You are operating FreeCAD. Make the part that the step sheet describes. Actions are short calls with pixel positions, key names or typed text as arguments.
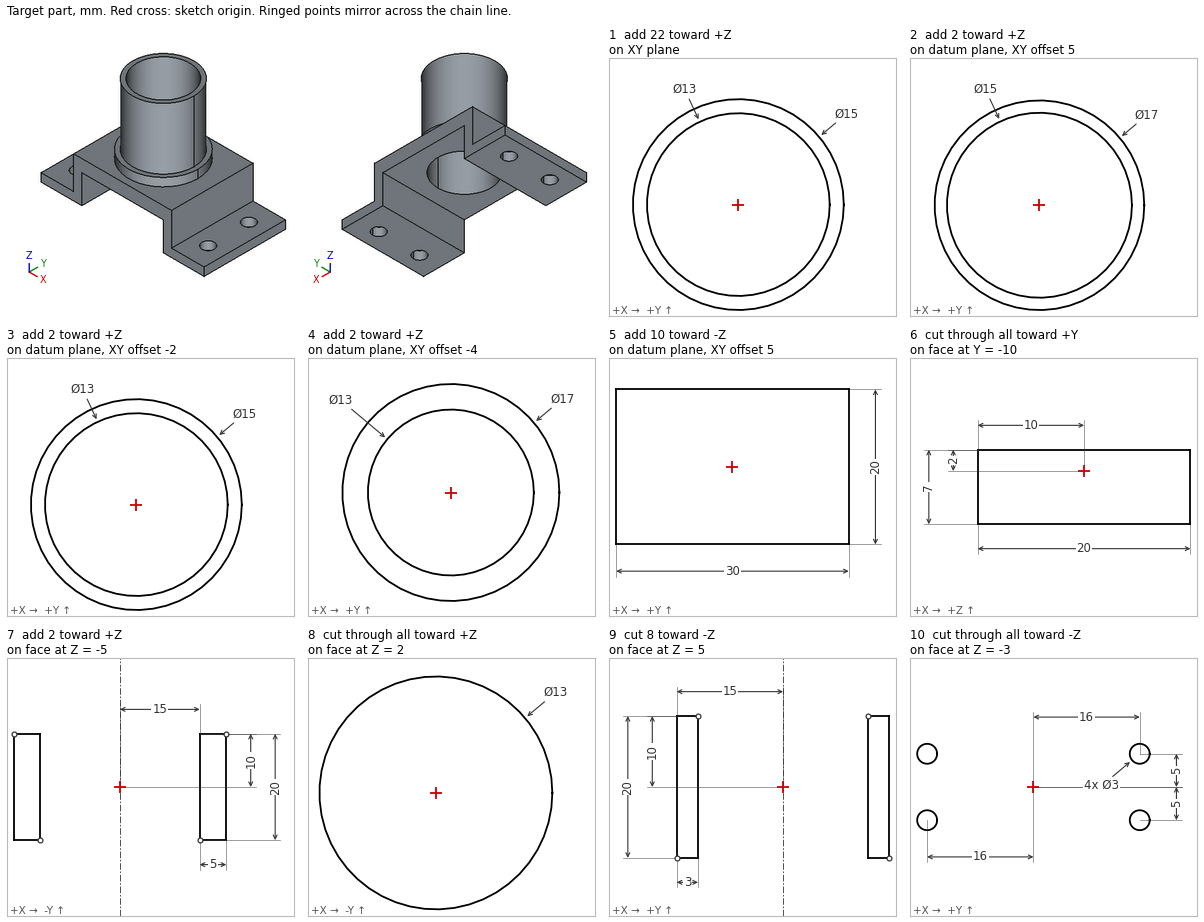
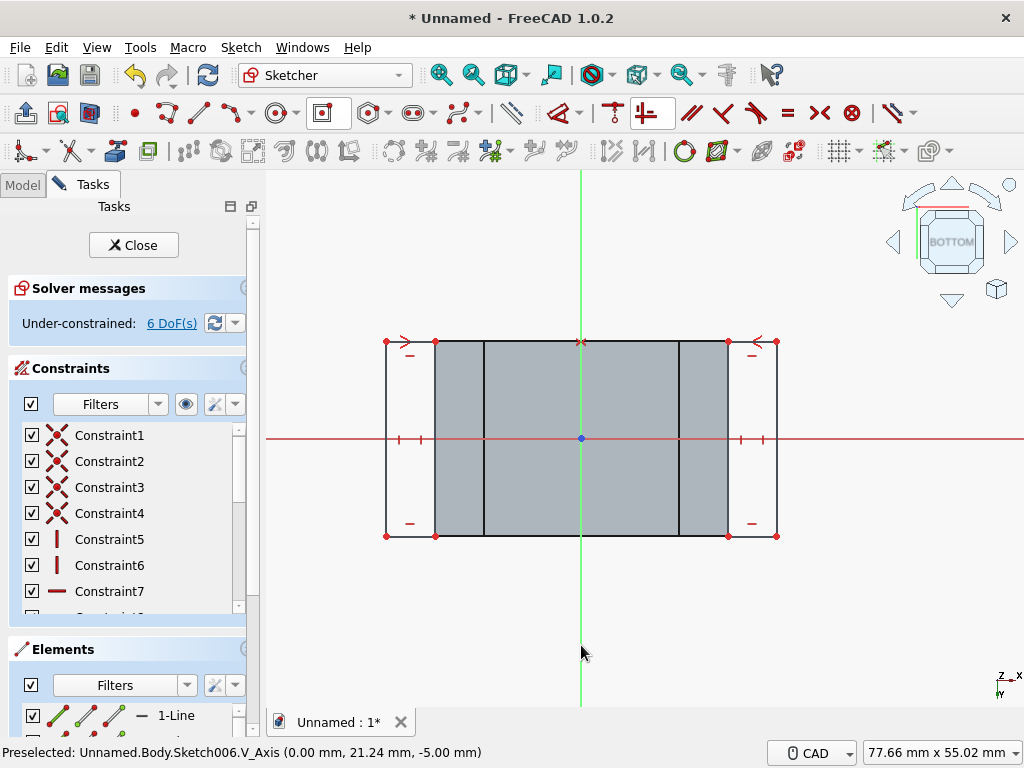
click(728, 537)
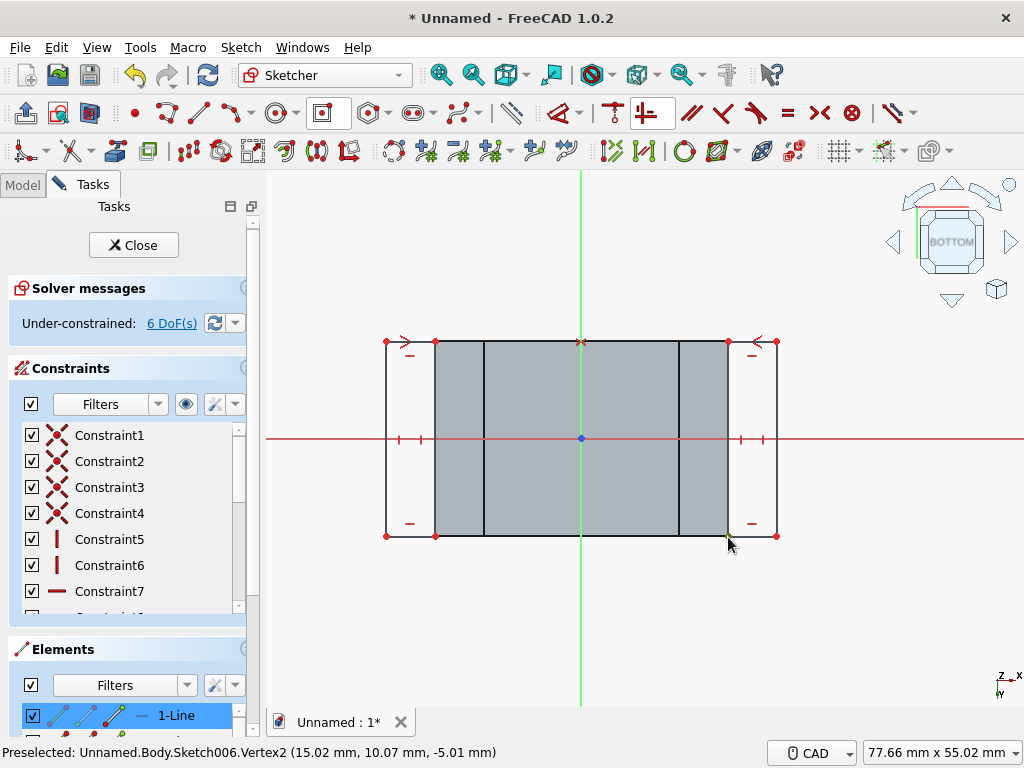
click(435, 537)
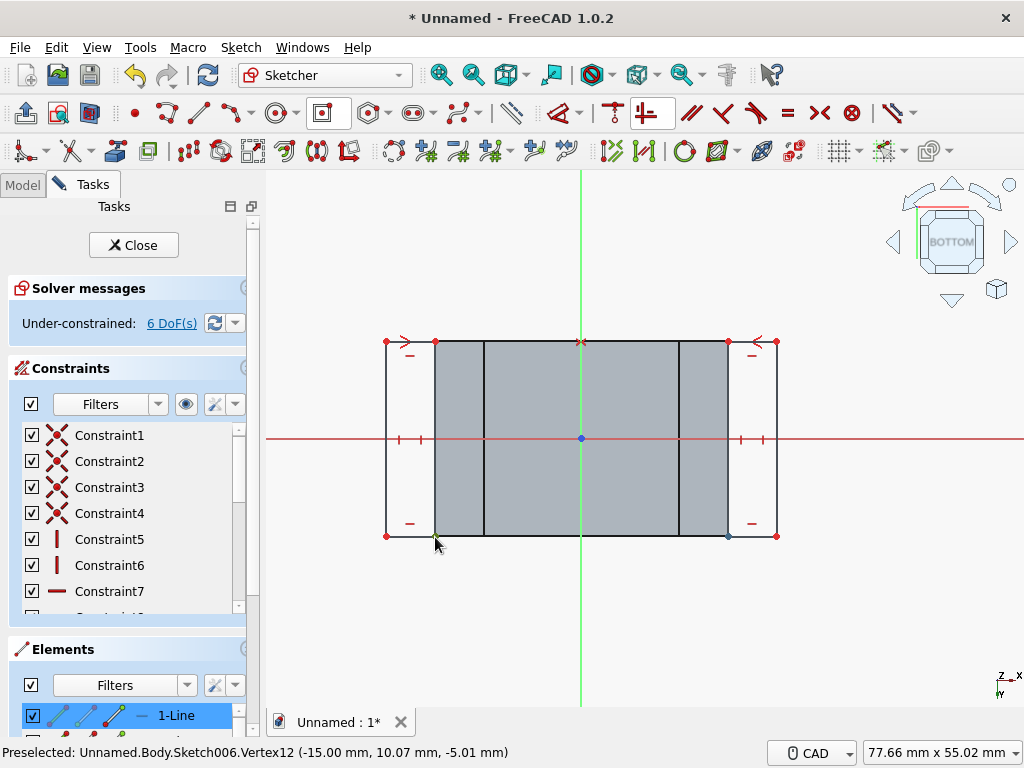
click(581, 645)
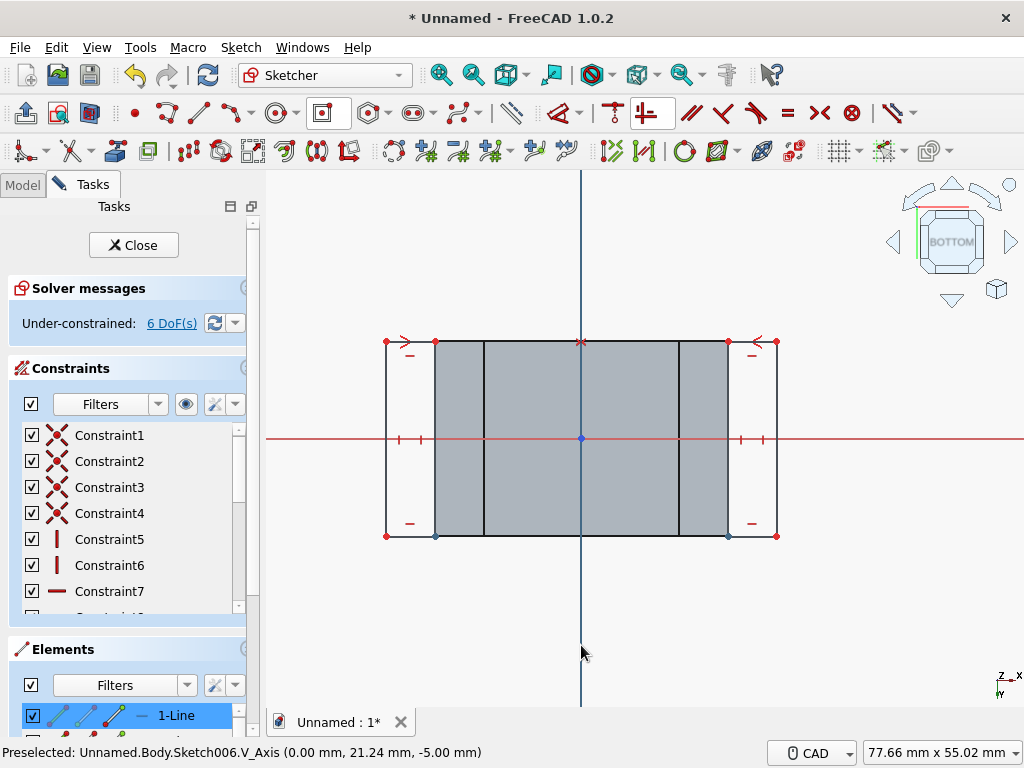
click(820, 114)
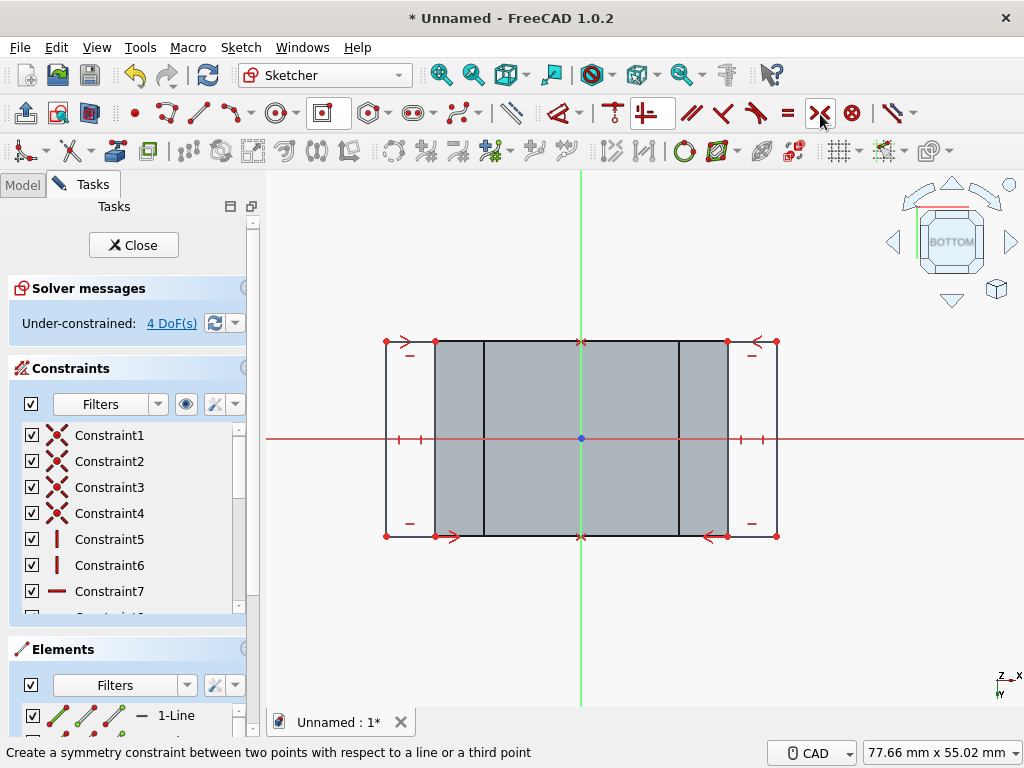
click(558, 114)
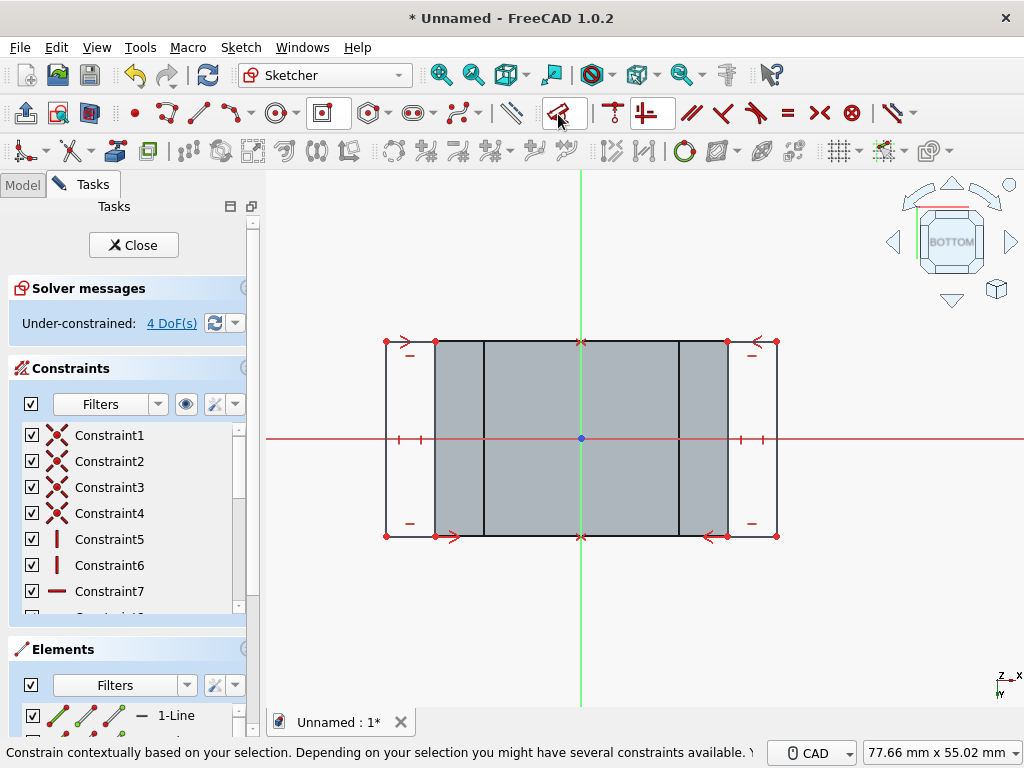
click(742, 537)
click(752, 571)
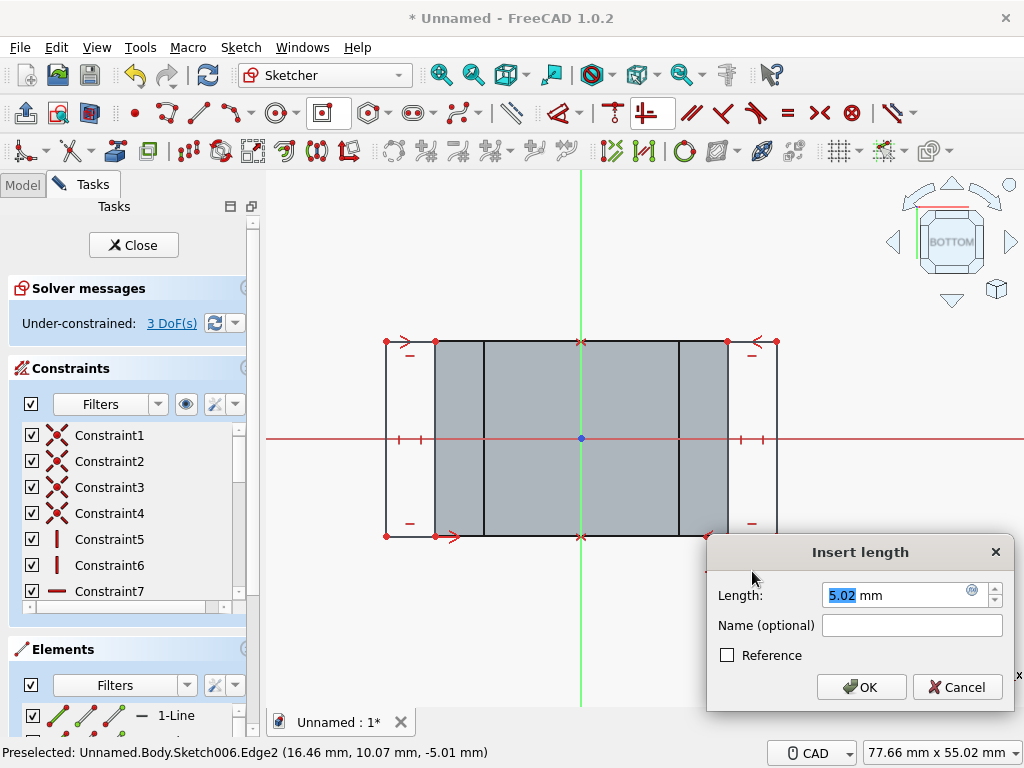
text(5)
key(Return)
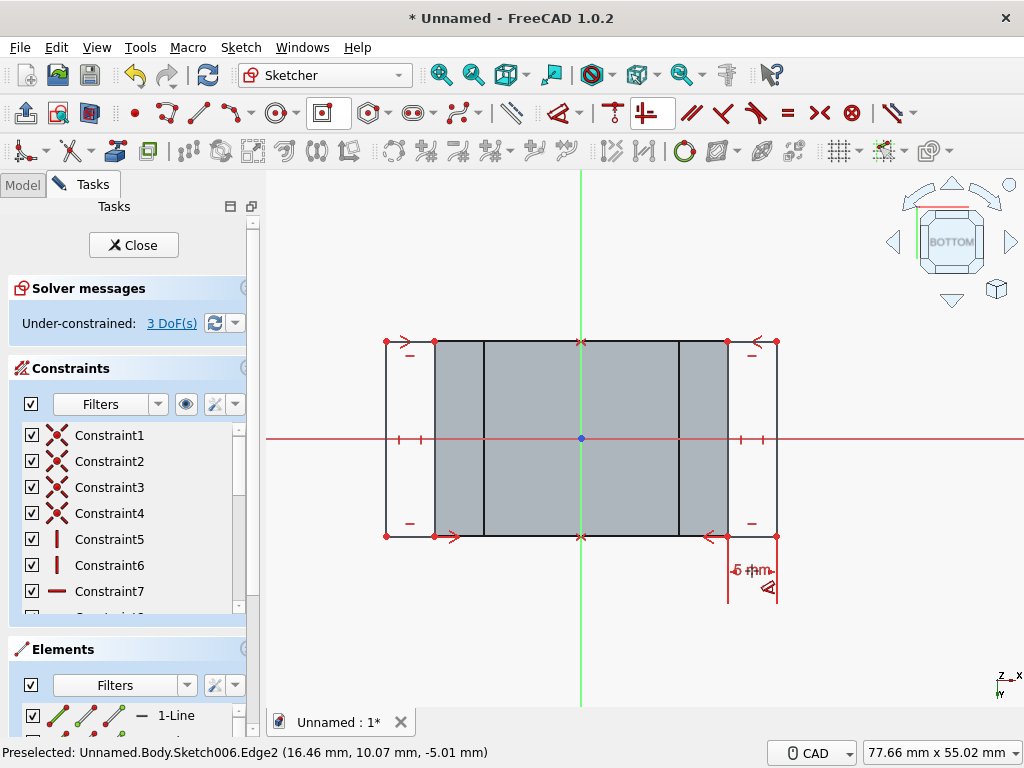
click(728, 400)
click(762, 395)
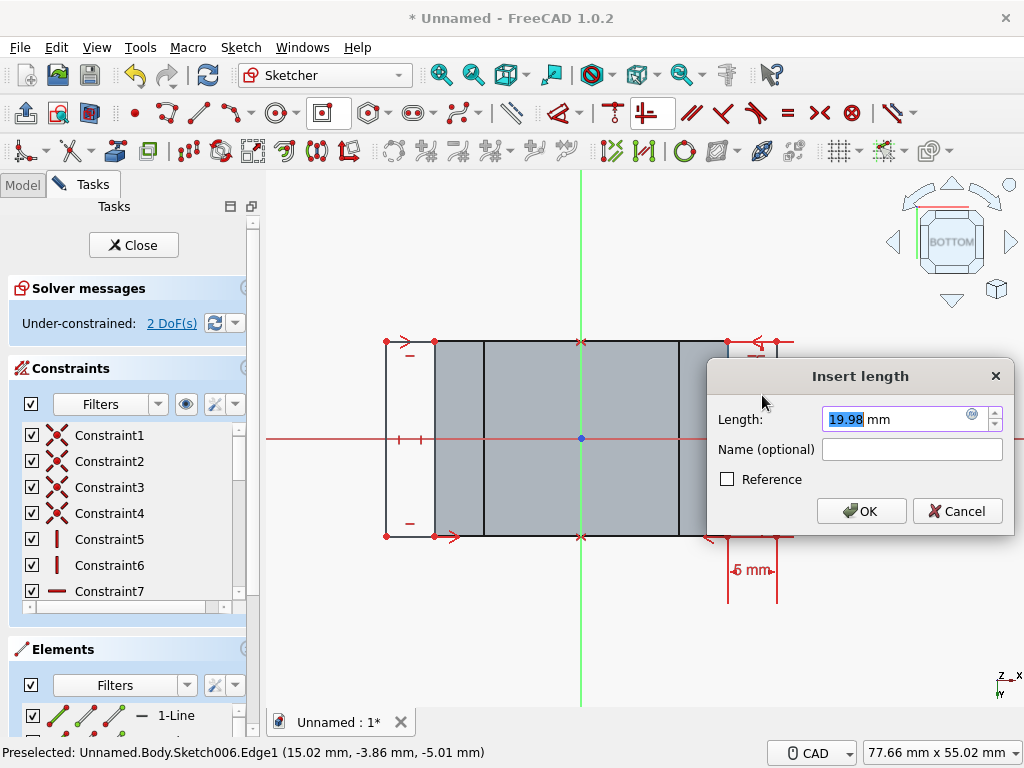
text(20)
key(Return)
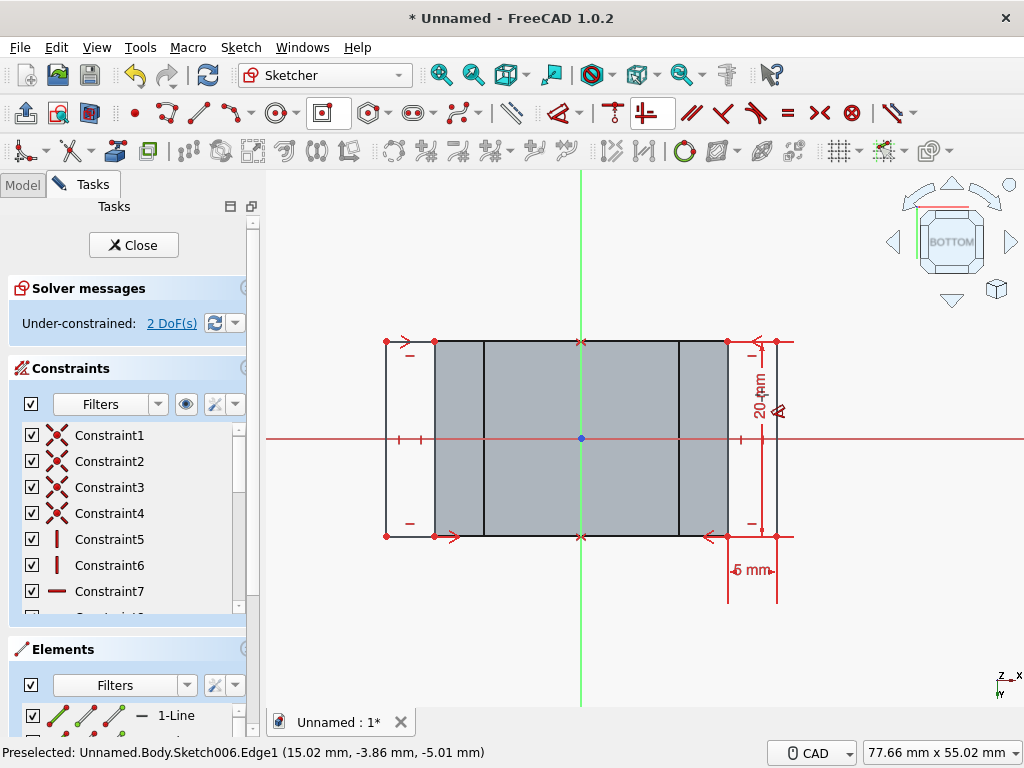
click(728, 342)
click(655, 308)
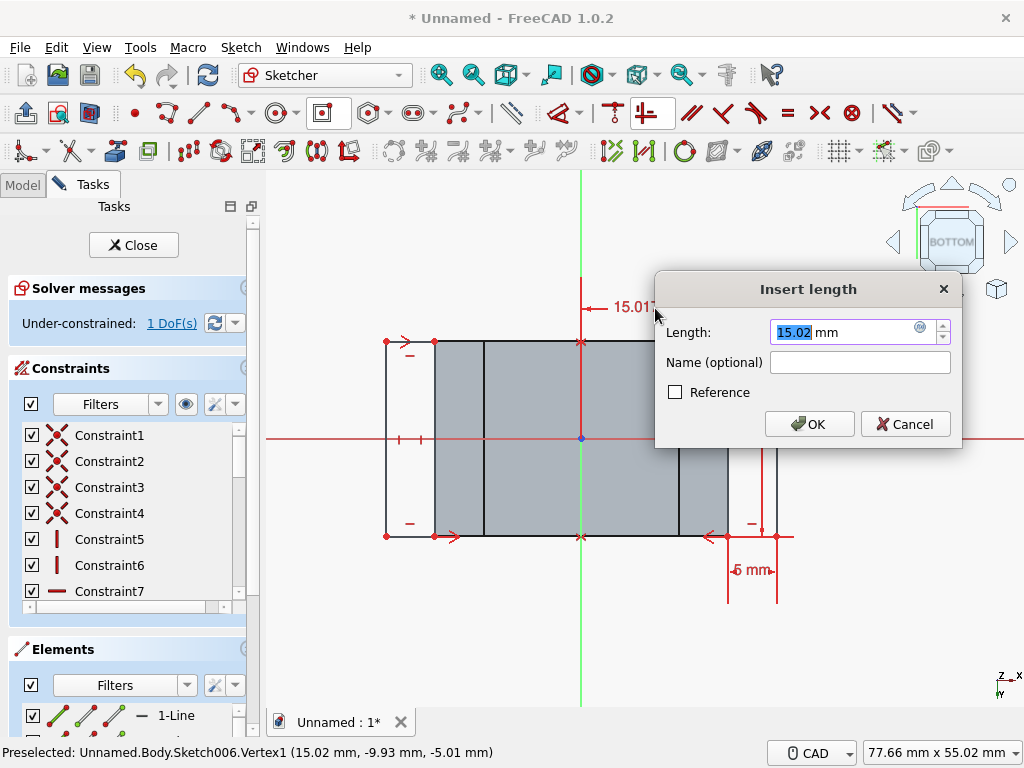
text(15)
key(Return)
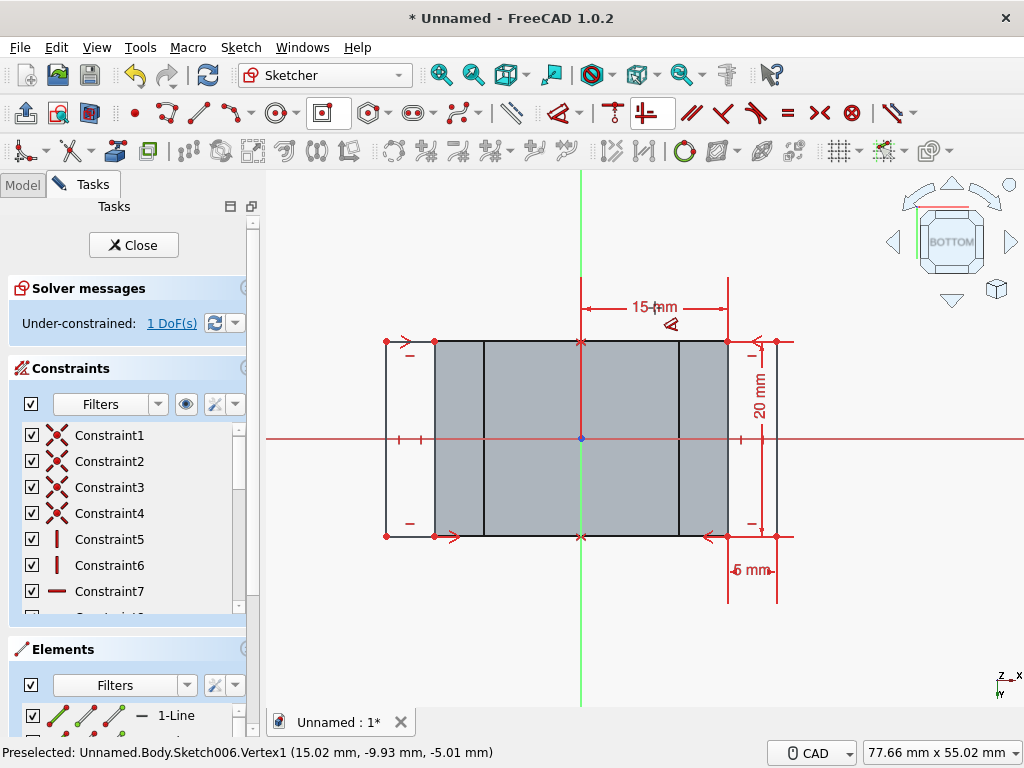
click(728, 342)
click(762, 368)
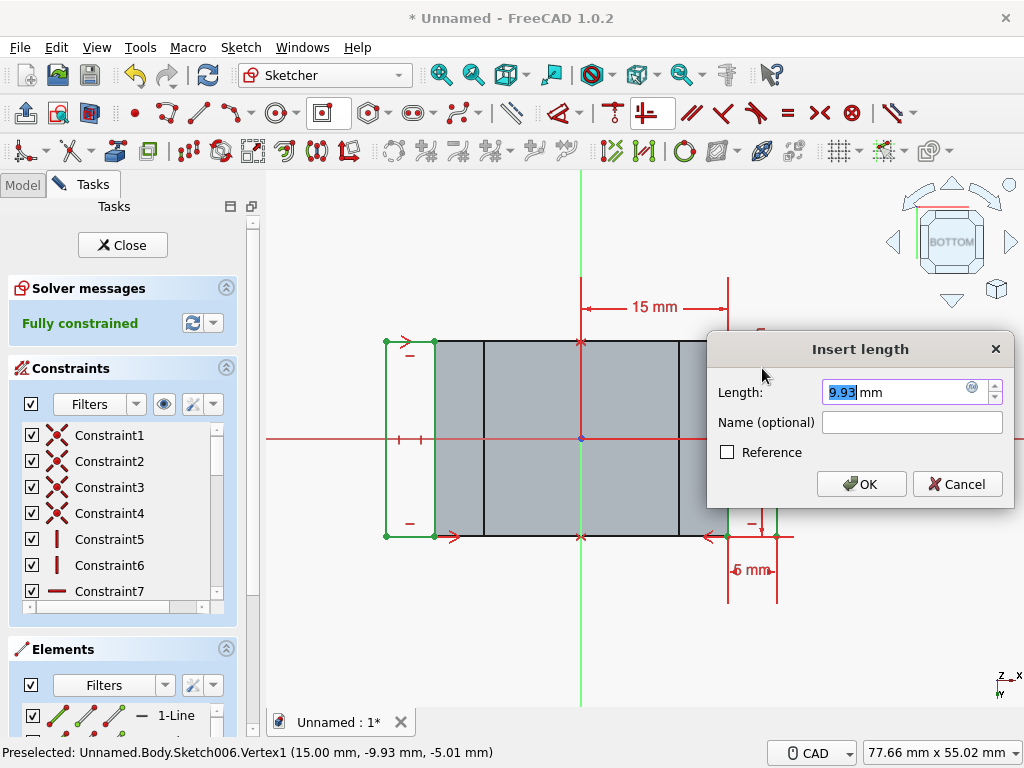
text(10)
key(Return)
key(Escape)